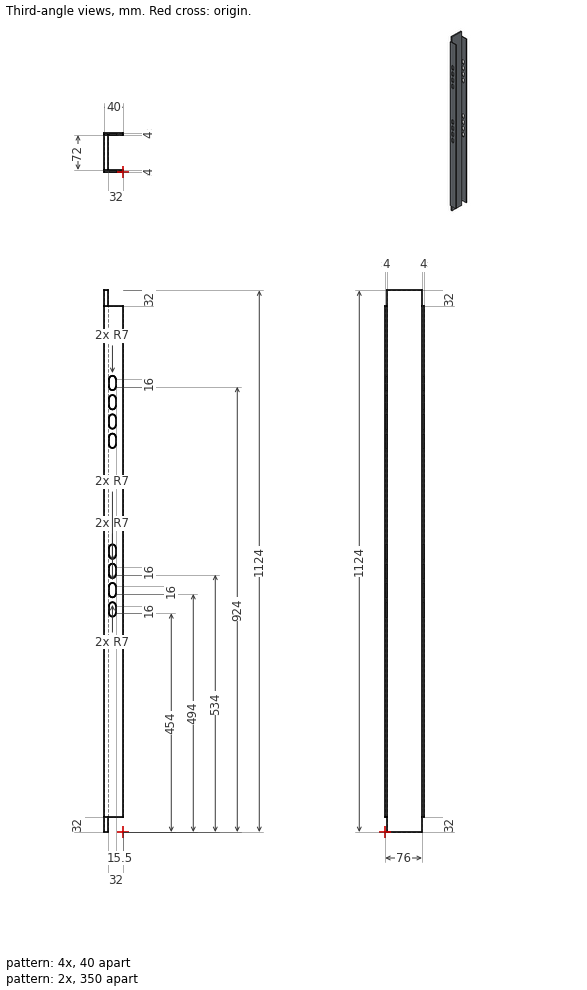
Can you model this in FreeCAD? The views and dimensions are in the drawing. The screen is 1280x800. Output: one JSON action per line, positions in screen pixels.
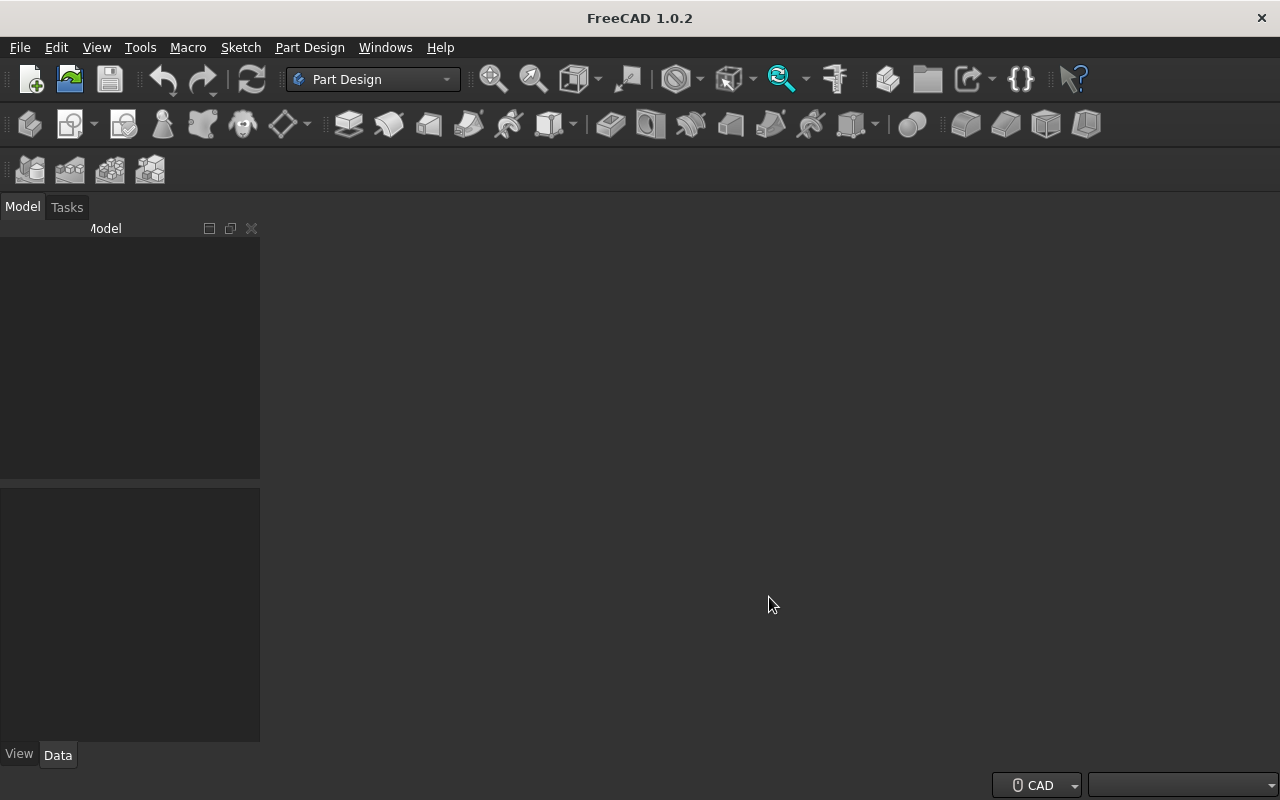
{"action": "key", "text": "ctrl+n"}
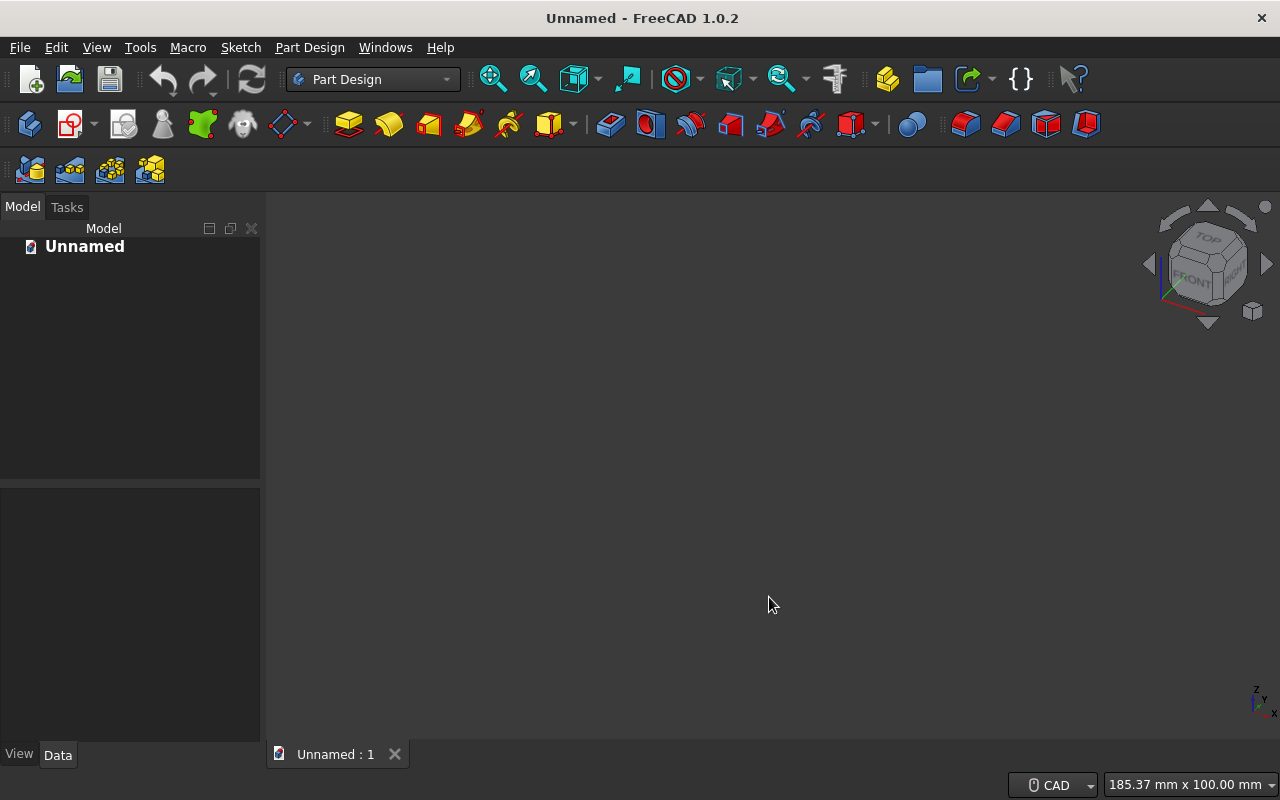
{"action": "left_click", "coordinate": [70, 124]}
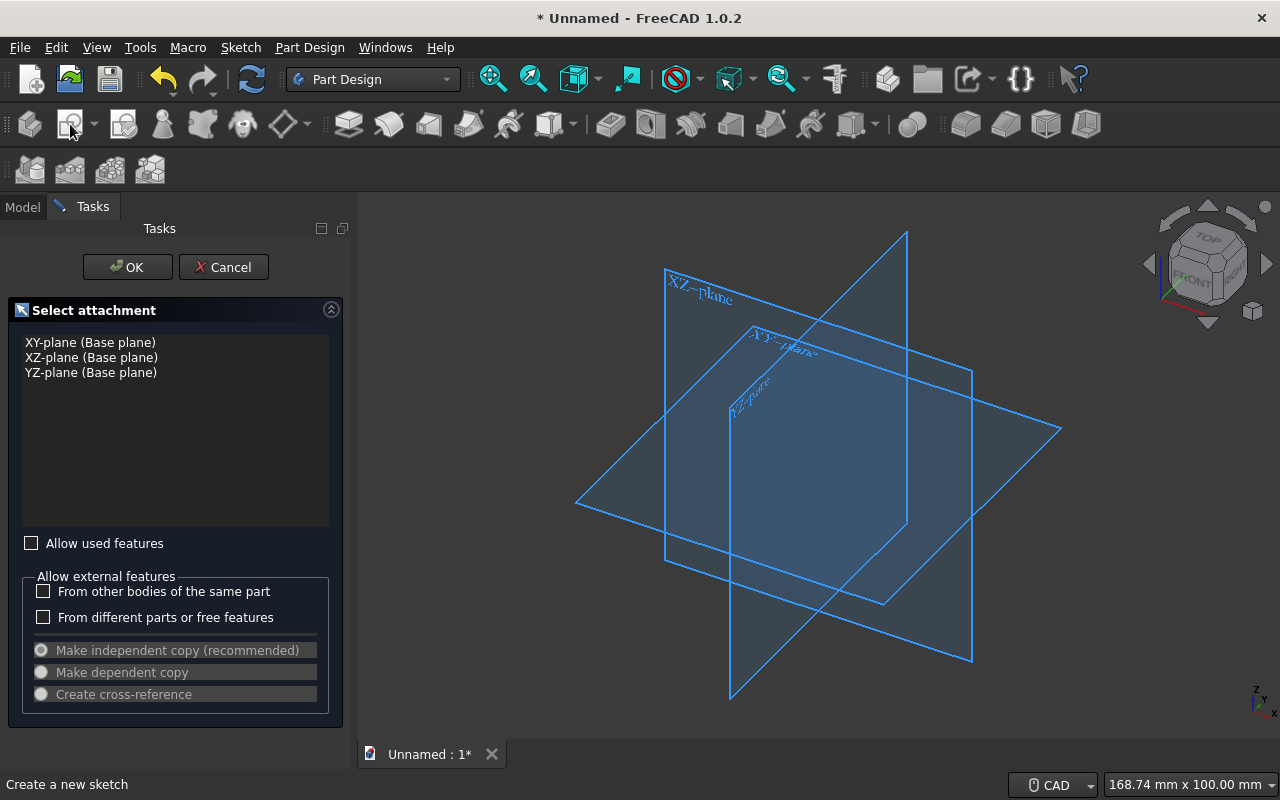
{"action": "left_click", "coordinate": [82, 342]}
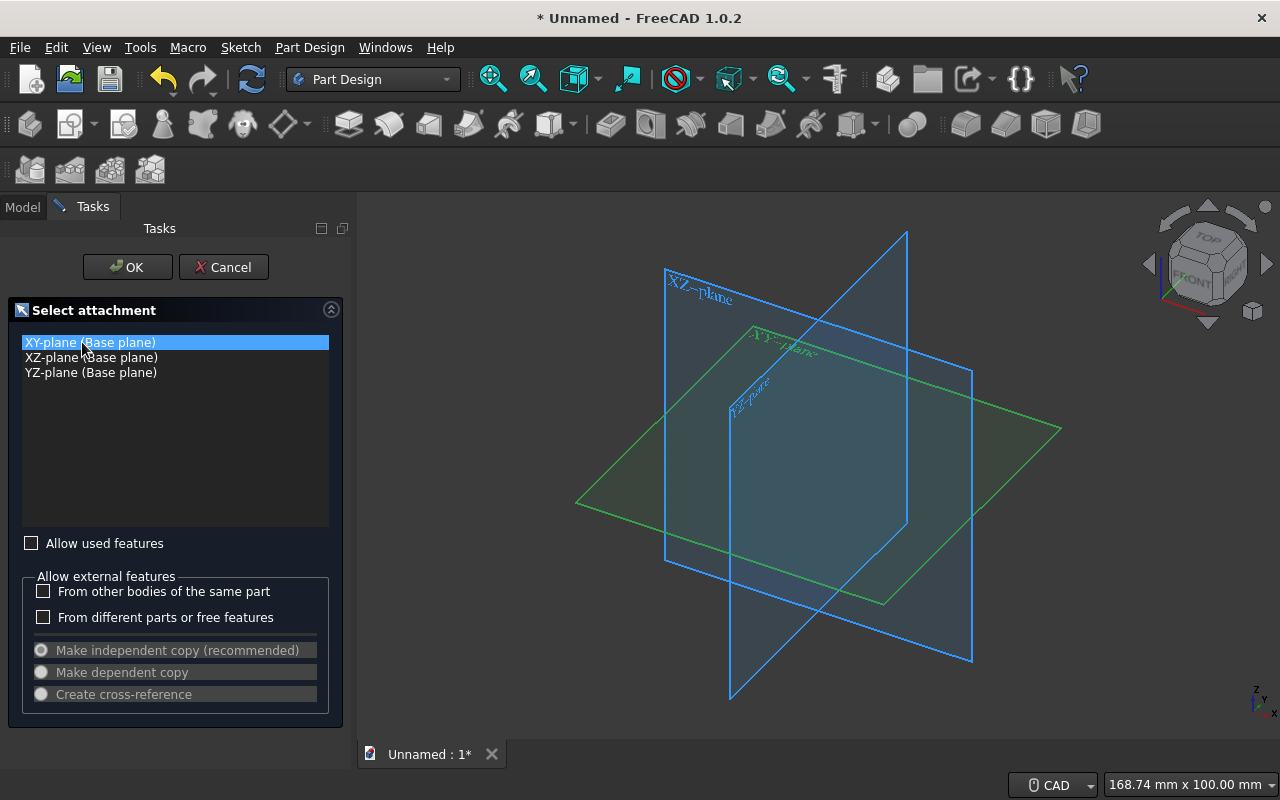
{"action": "left_click", "coordinate": [128, 267]}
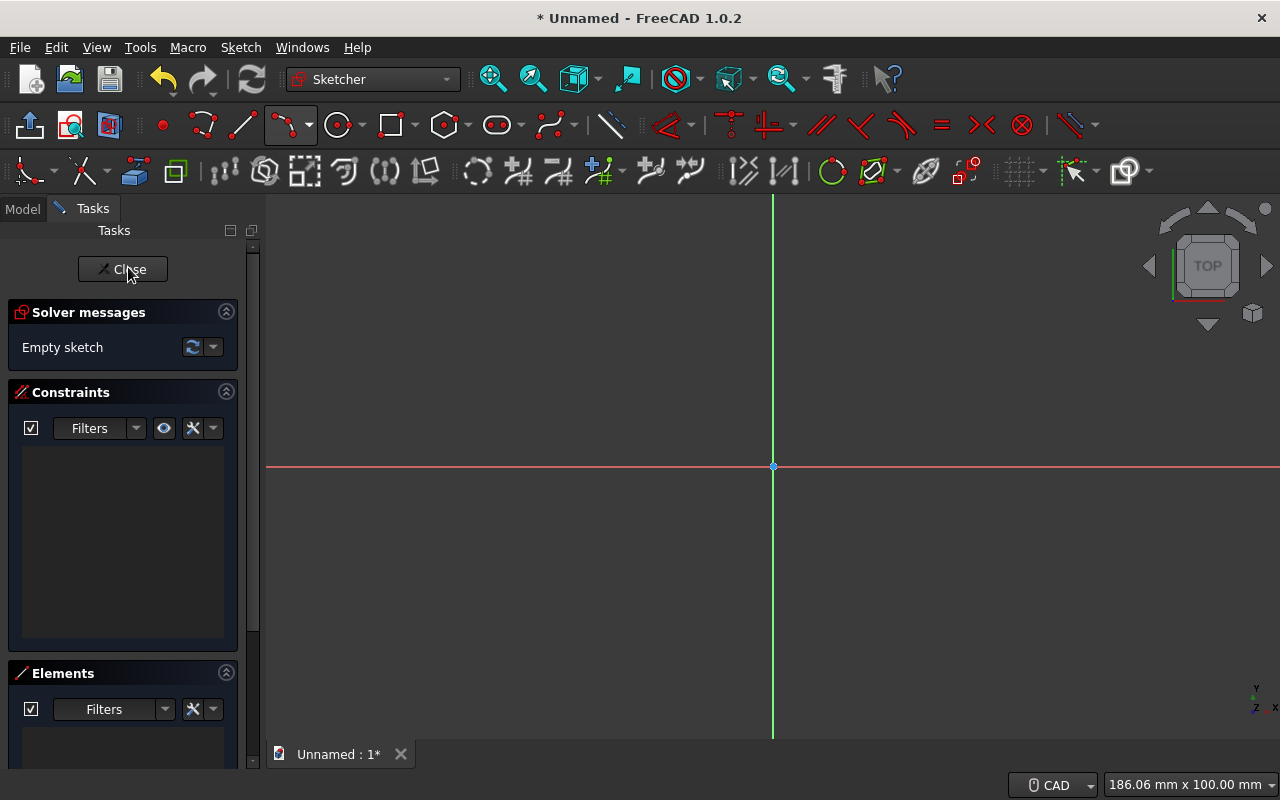
{"action": "scroll", "coordinate": [787, 711], "scroll_direction": "down", "scroll_amount": 2}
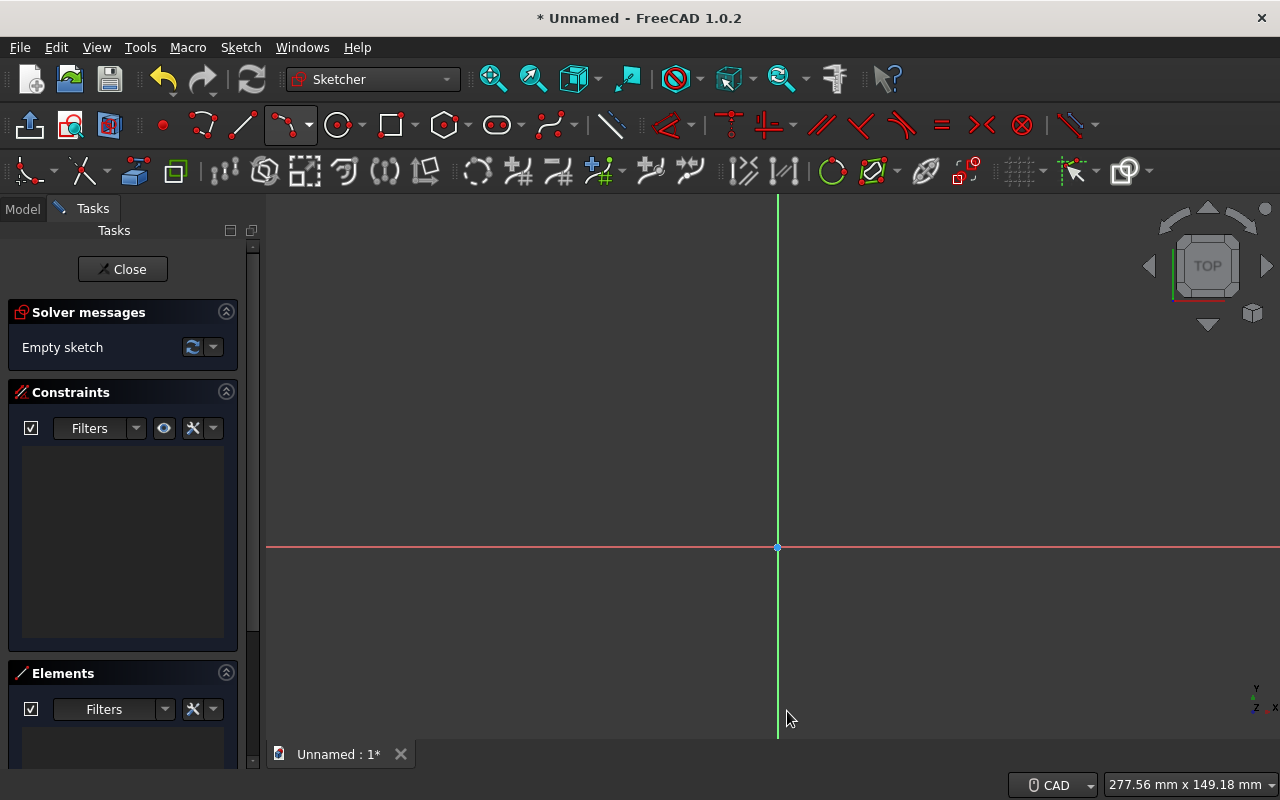
{"action": "left_click", "coordinate": [204, 126]}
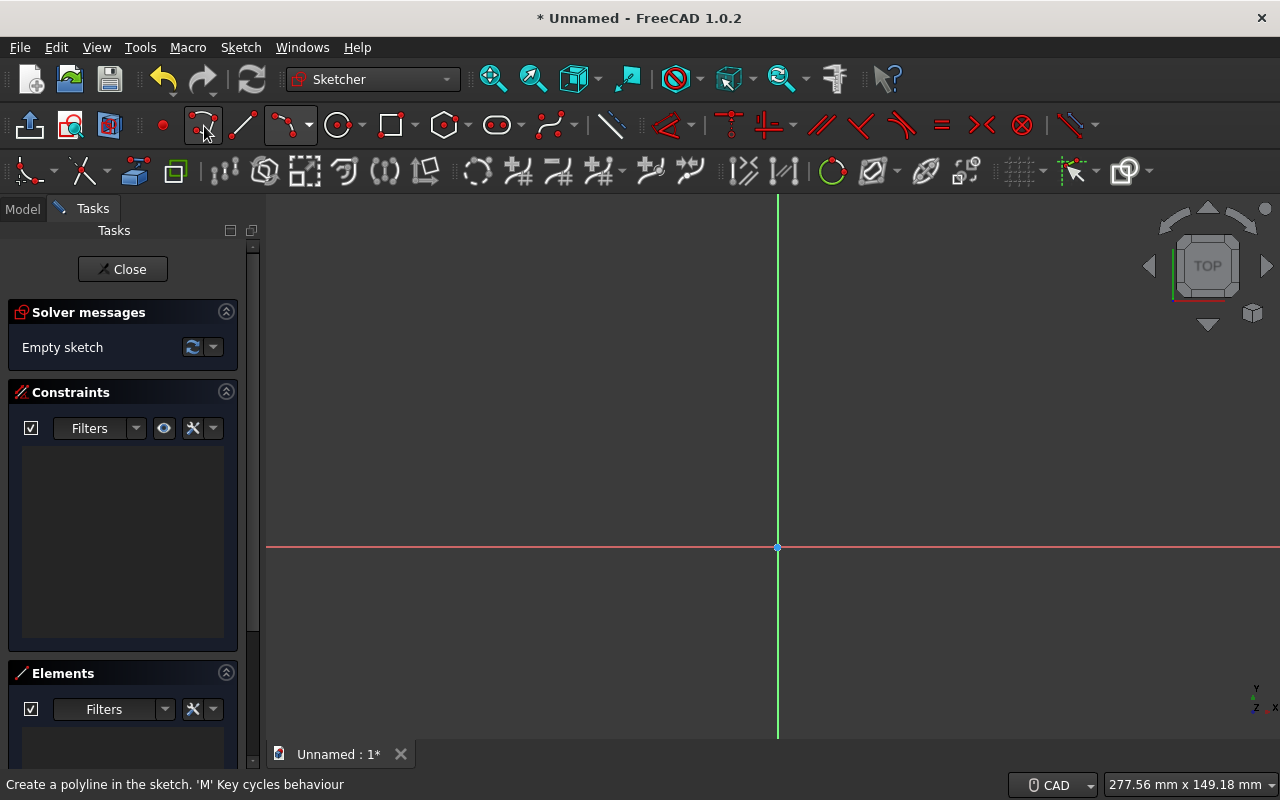
{"action": "left_click", "coordinate": [778, 547]}
{"action": "left_click", "coordinate": [769, 533]}
{"action": "left_click", "coordinate": [661, 533]}
{"action": "left_click", "coordinate": [661, 270]}
{"action": "left_click", "coordinate": [778, 270]}
{"action": "left_click", "coordinate": [769, 255]}
{"action": "left_click", "coordinate": [632, 255]}
{"action": "left_click", "coordinate": [632, 538]}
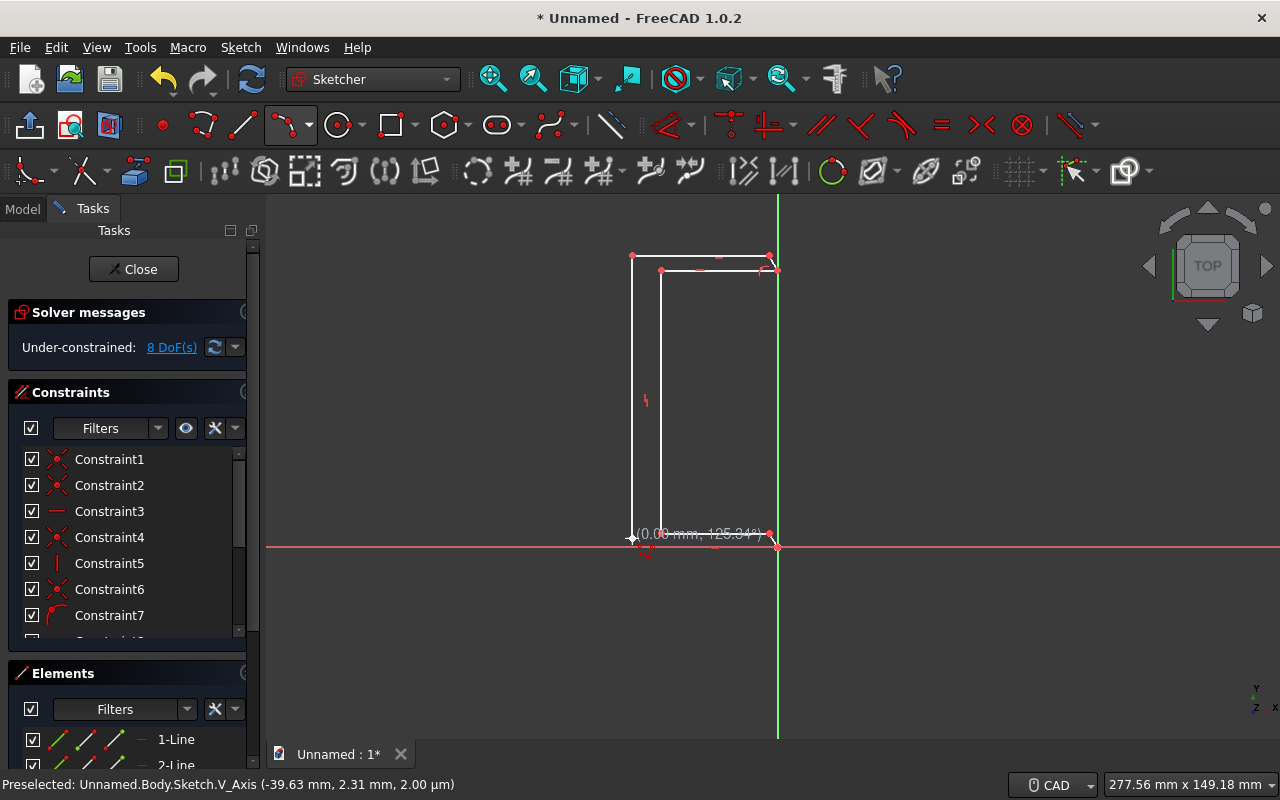
{"action": "scroll", "coordinate": [778, 547], "scroll_direction": "up", "scroll_amount": 4}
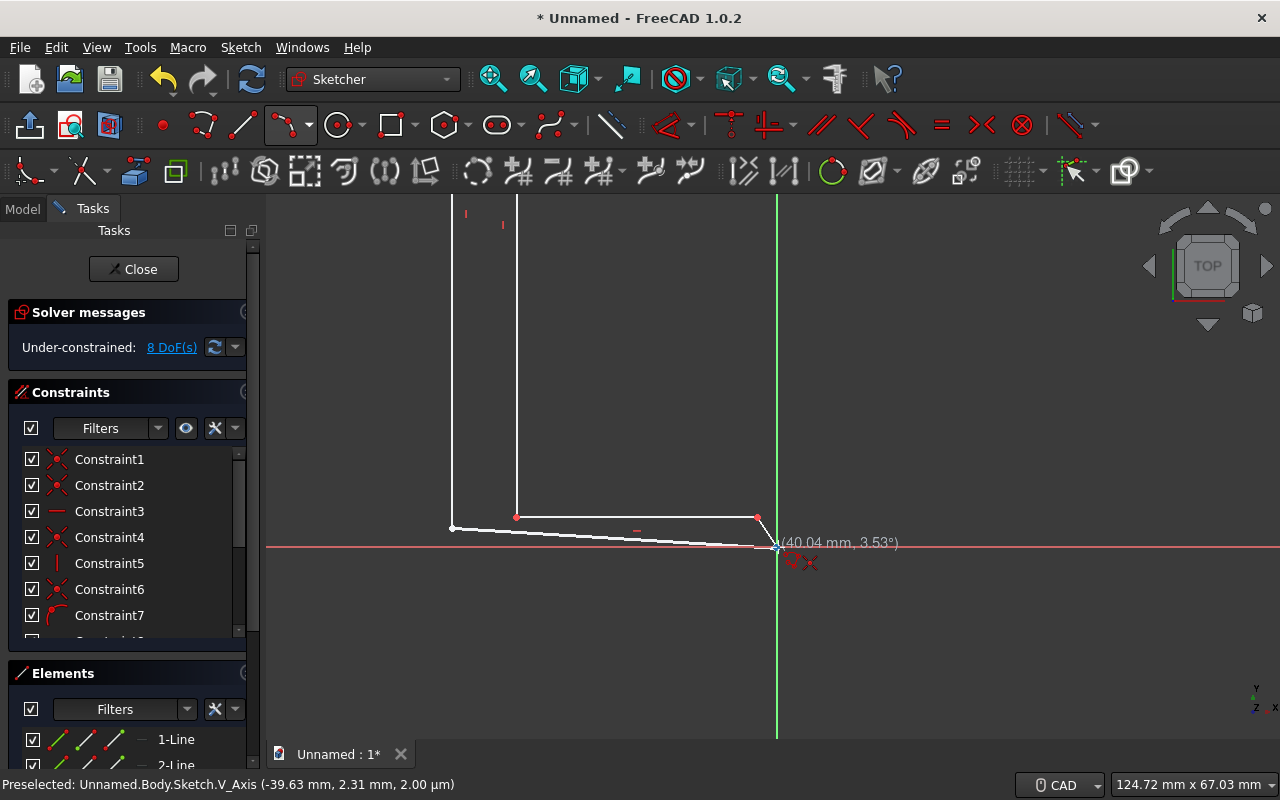
{"action": "left_click", "coordinate": [777, 547]}
{"action": "key", "text": "Escape"}
{"action": "key", "text": "Escape"}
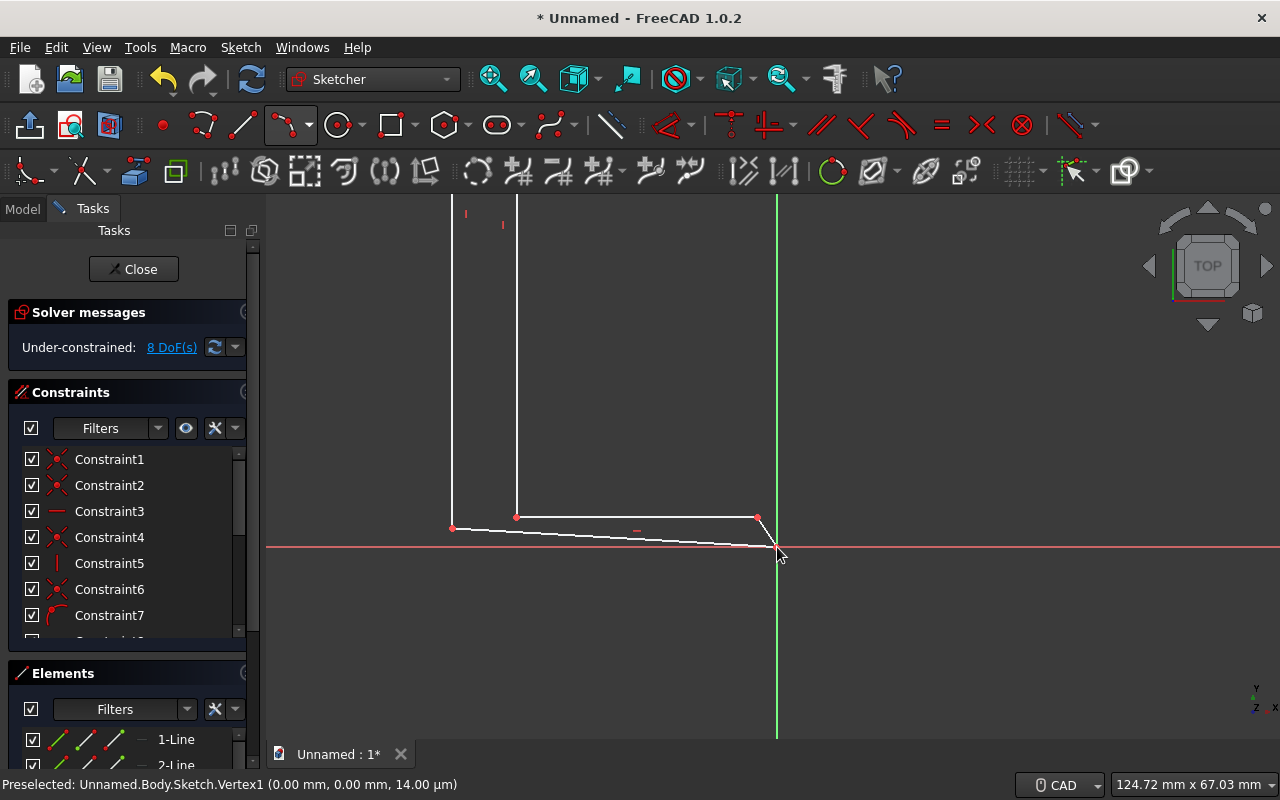
{"action": "scroll", "coordinate": [763, 526], "scroll_direction": "up", "scroll_amount": 2}